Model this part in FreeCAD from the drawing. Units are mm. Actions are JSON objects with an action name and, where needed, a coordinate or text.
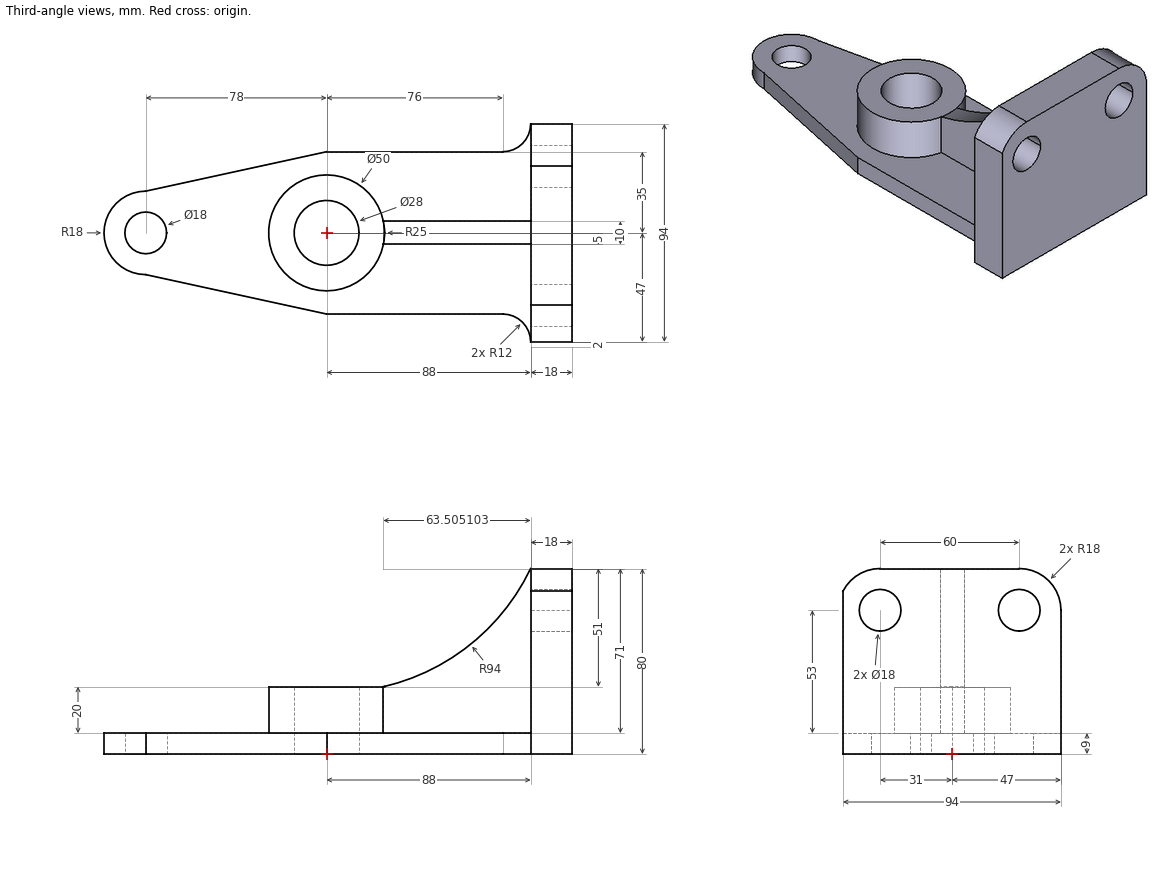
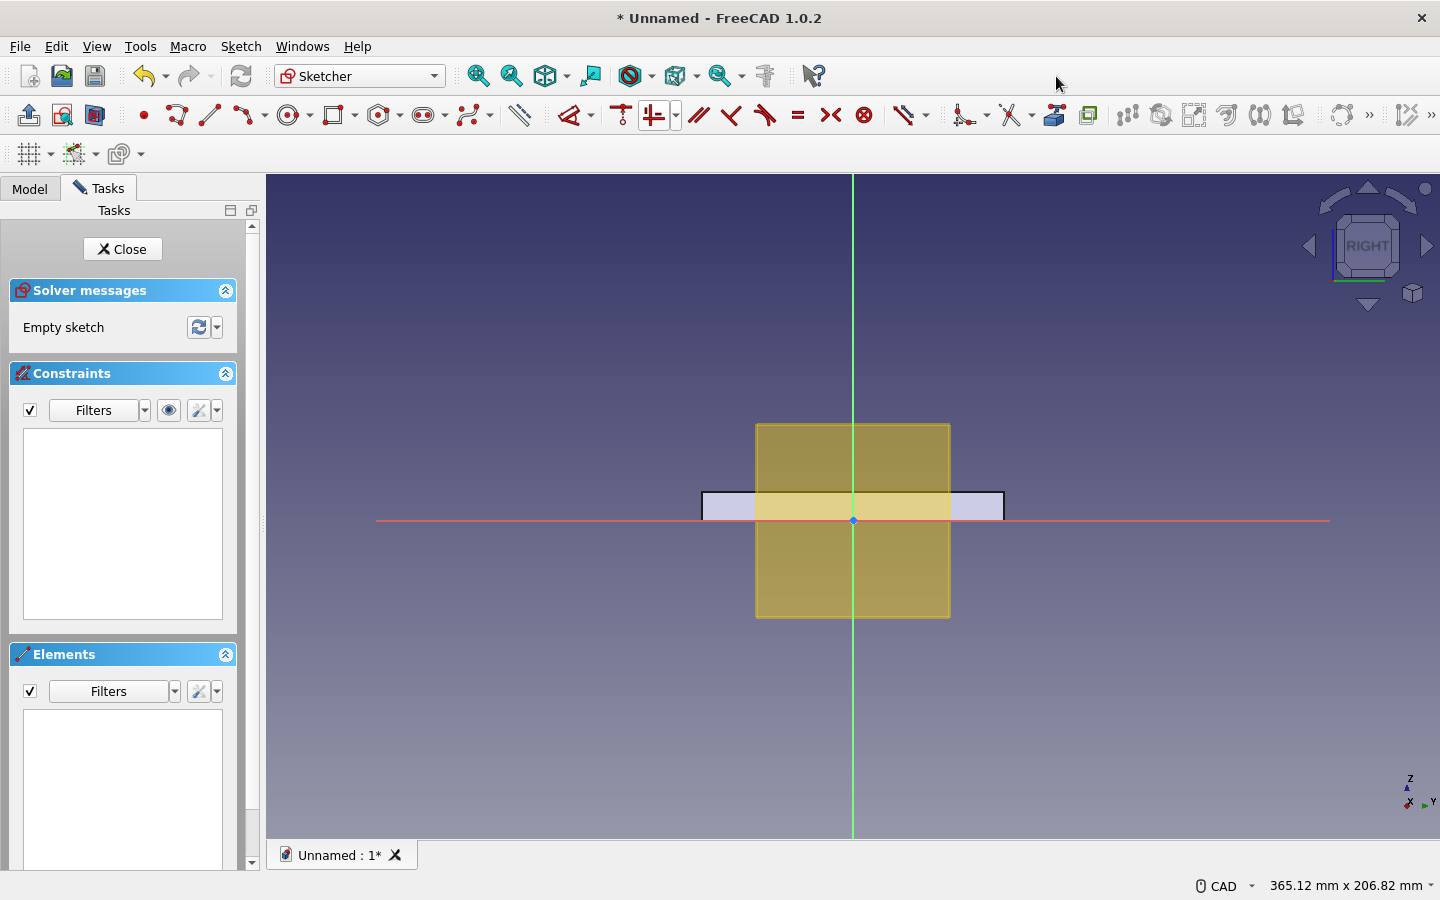
{"action": "scroll", "coordinate": [929, 254], "scroll_direction": "up", "scroll_amount": 3}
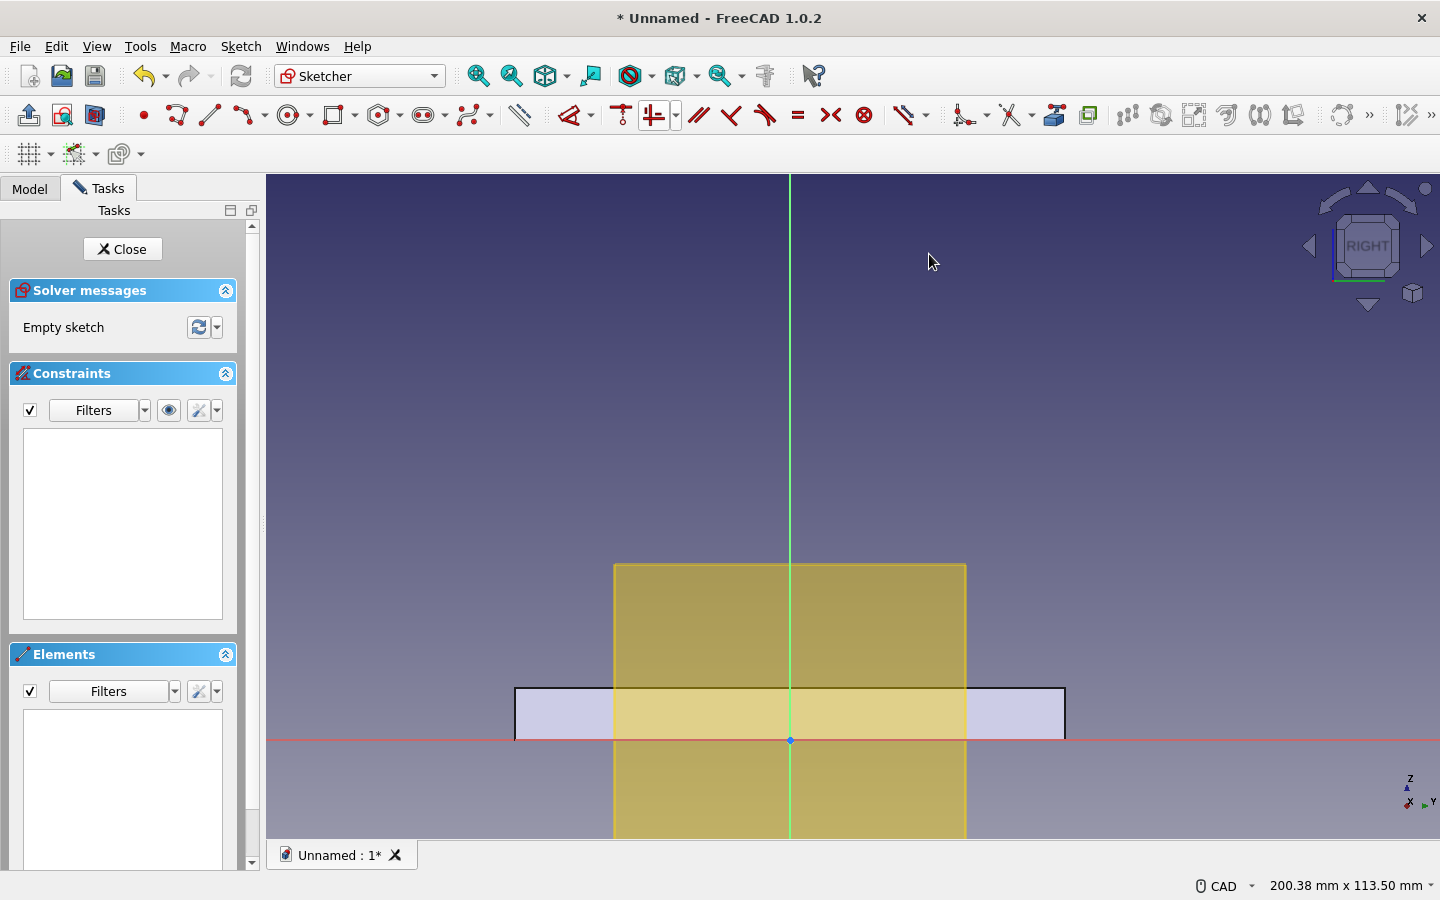
{"action": "left_click", "coordinate": [210, 116]}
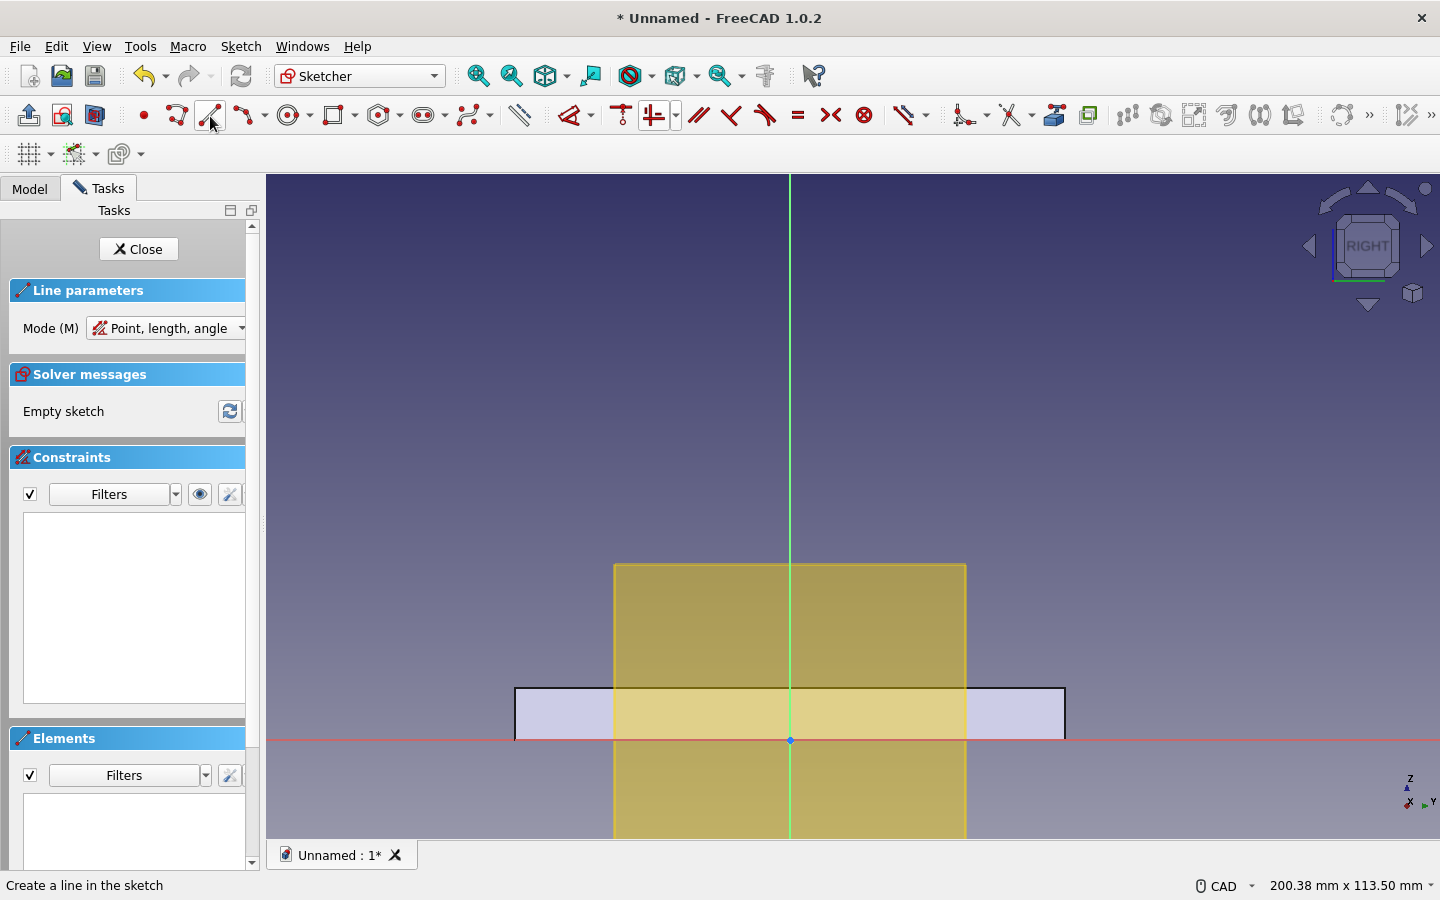
{"action": "left_click", "coordinate": [960, 272]}
{"action": "left_click", "coordinate": [608, 272]}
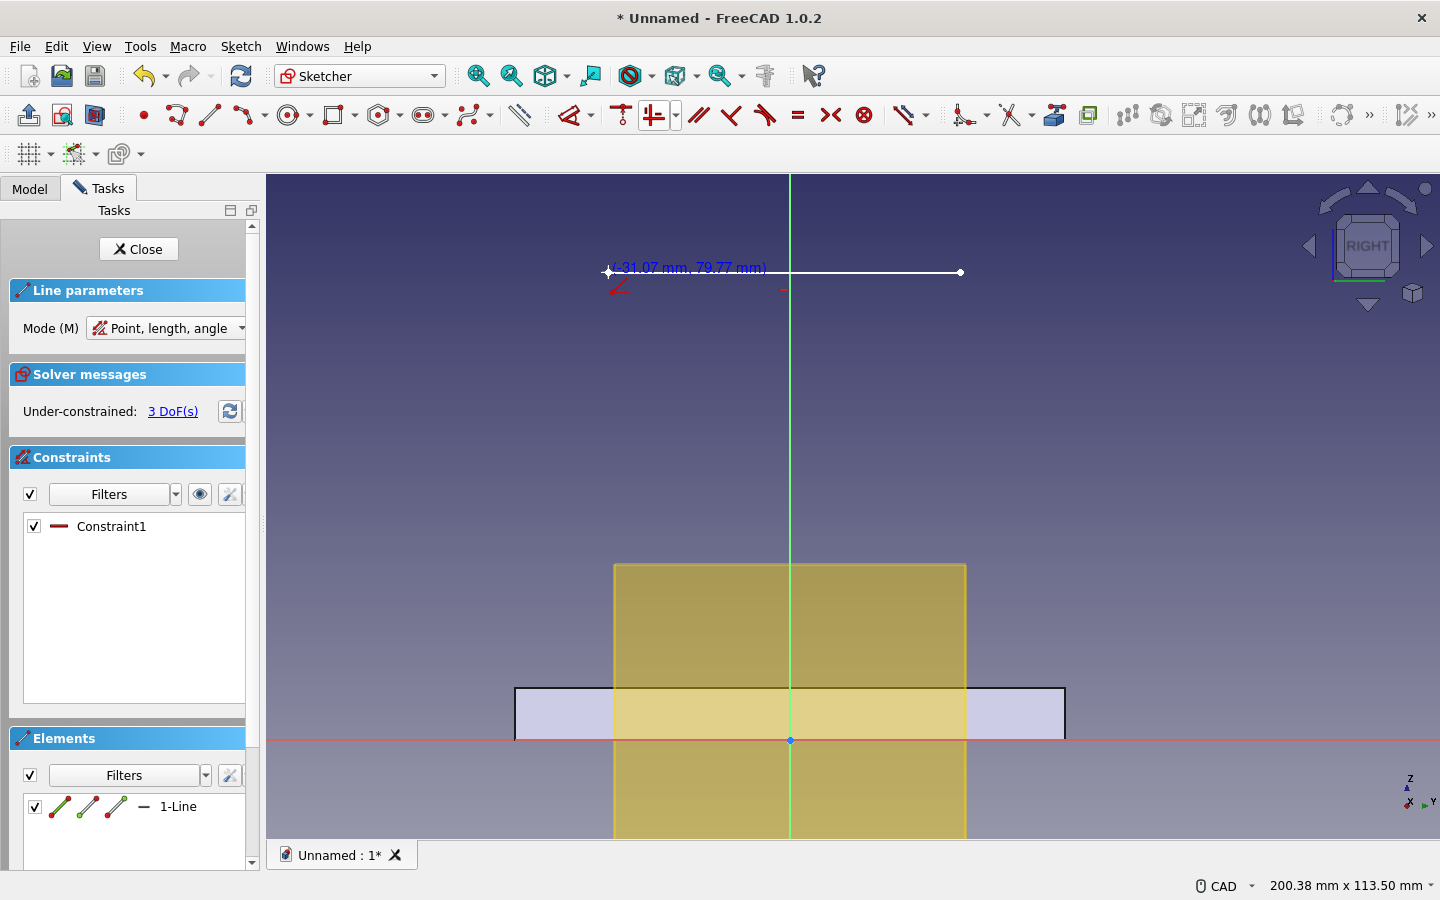
{"action": "left_click", "coordinate": [177, 116]}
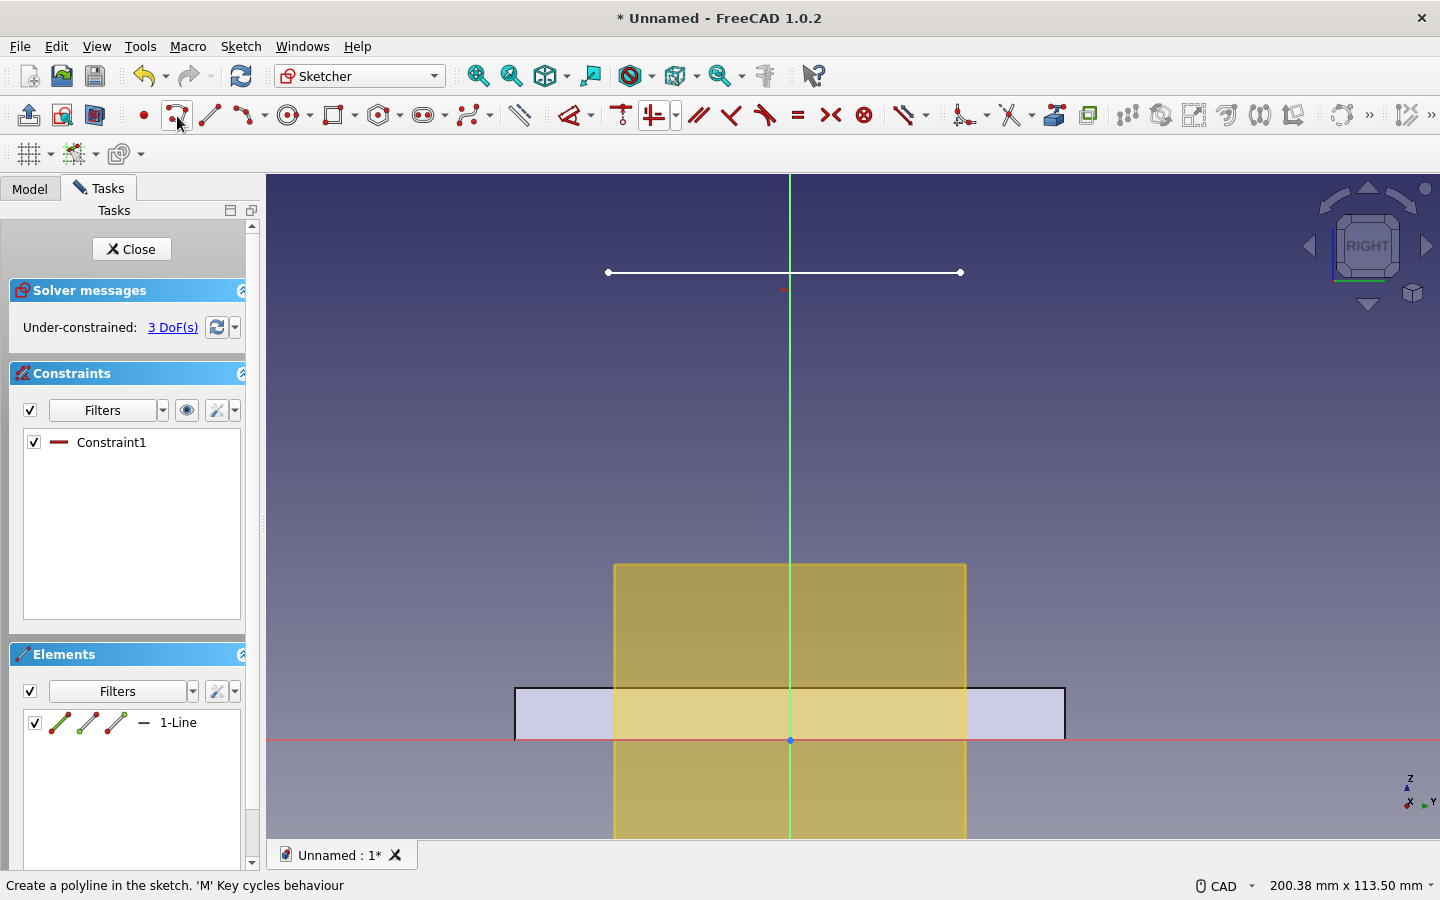
{"action": "left_click", "coordinate": [503, 377]}
{"action": "left_click", "coordinate": [503, 688]}
{"action": "left_click", "coordinate": [1065, 688]}
{"action": "left_click", "coordinate": [1065, 377]}
{"action": "right_click", "coordinate": [1065, 377]}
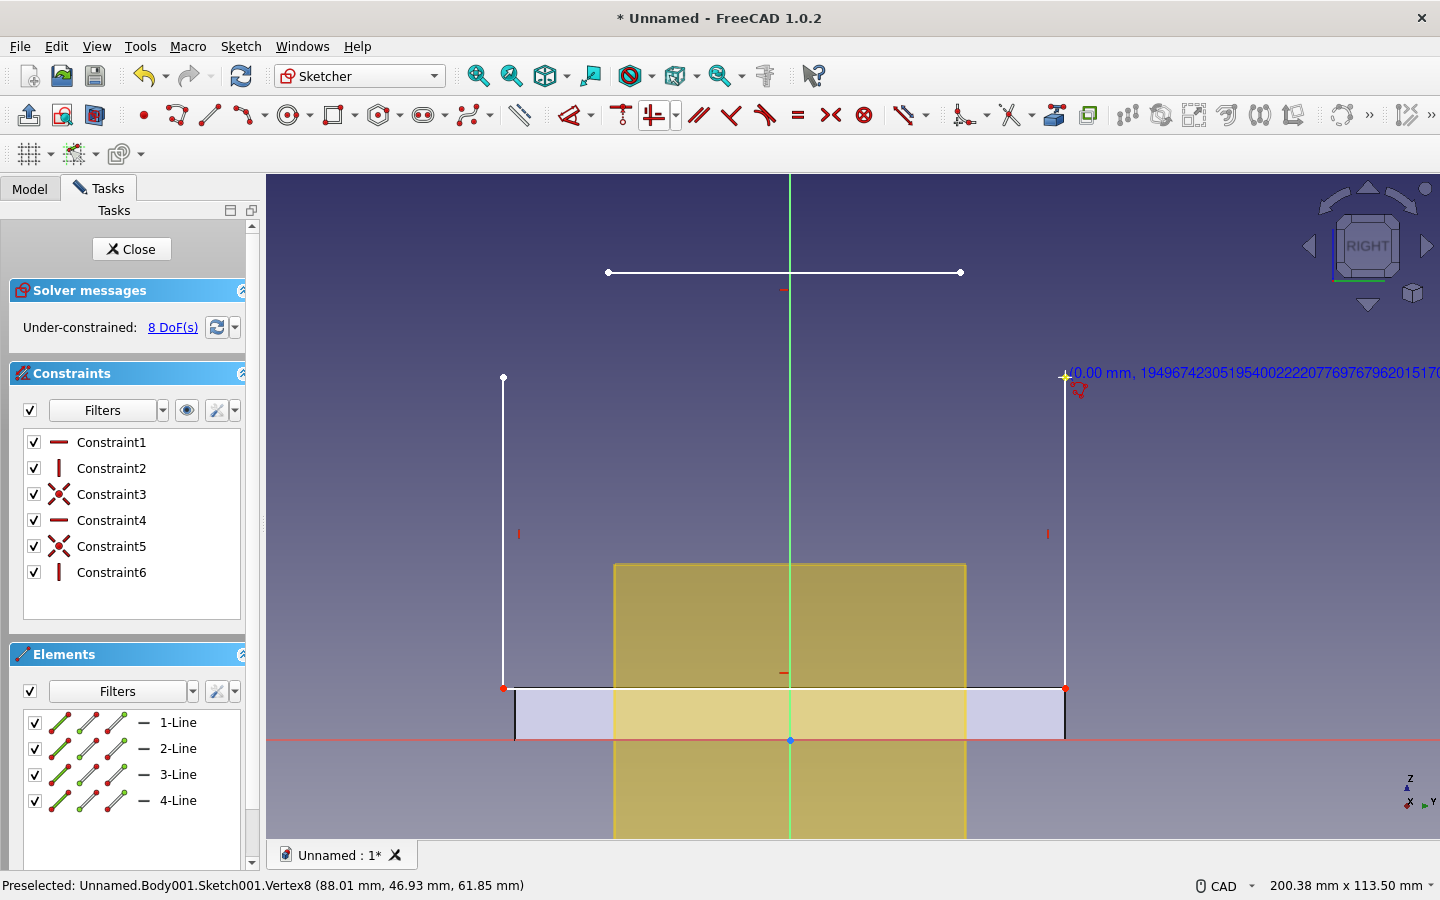
{"action": "left_click", "coordinate": [242, 116]}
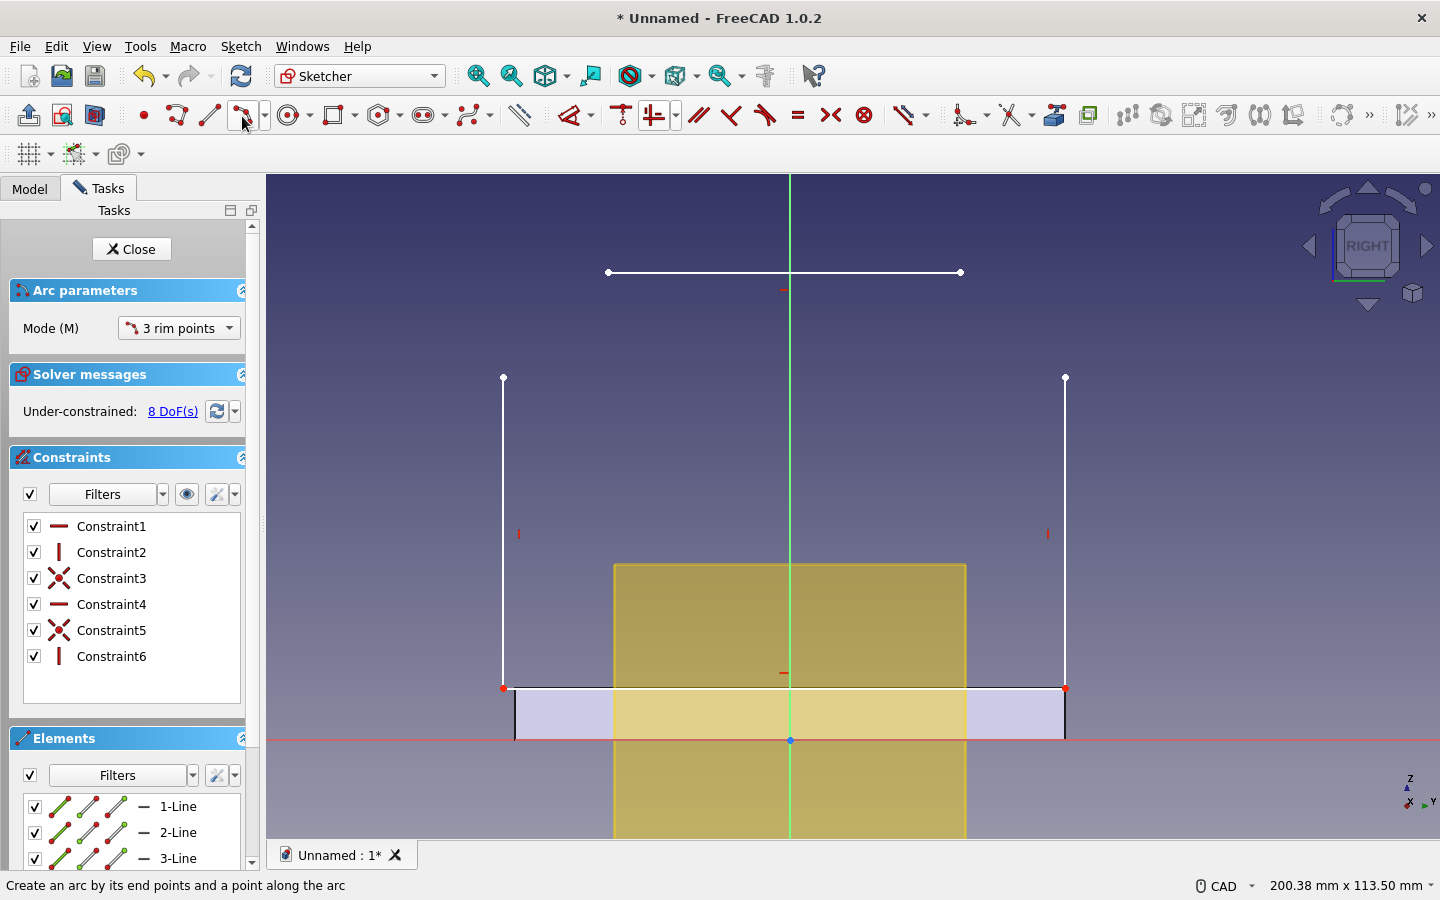
{"action": "left_click", "coordinate": [608, 273]}
{"action": "left_click", "coordinate": [503, 378]}
{"action": "left_click", "coordinate": [534, 303]}